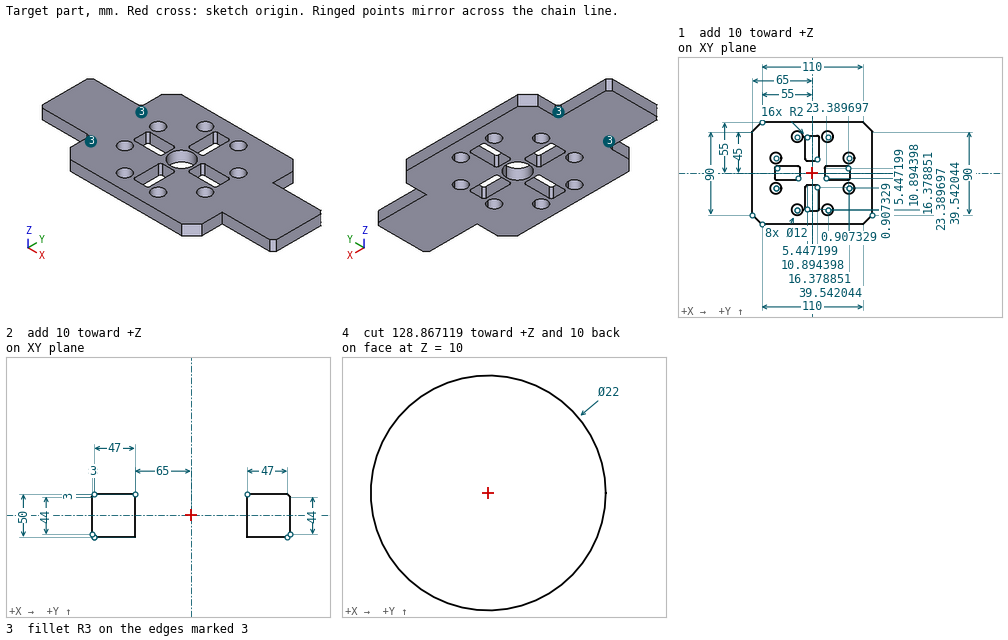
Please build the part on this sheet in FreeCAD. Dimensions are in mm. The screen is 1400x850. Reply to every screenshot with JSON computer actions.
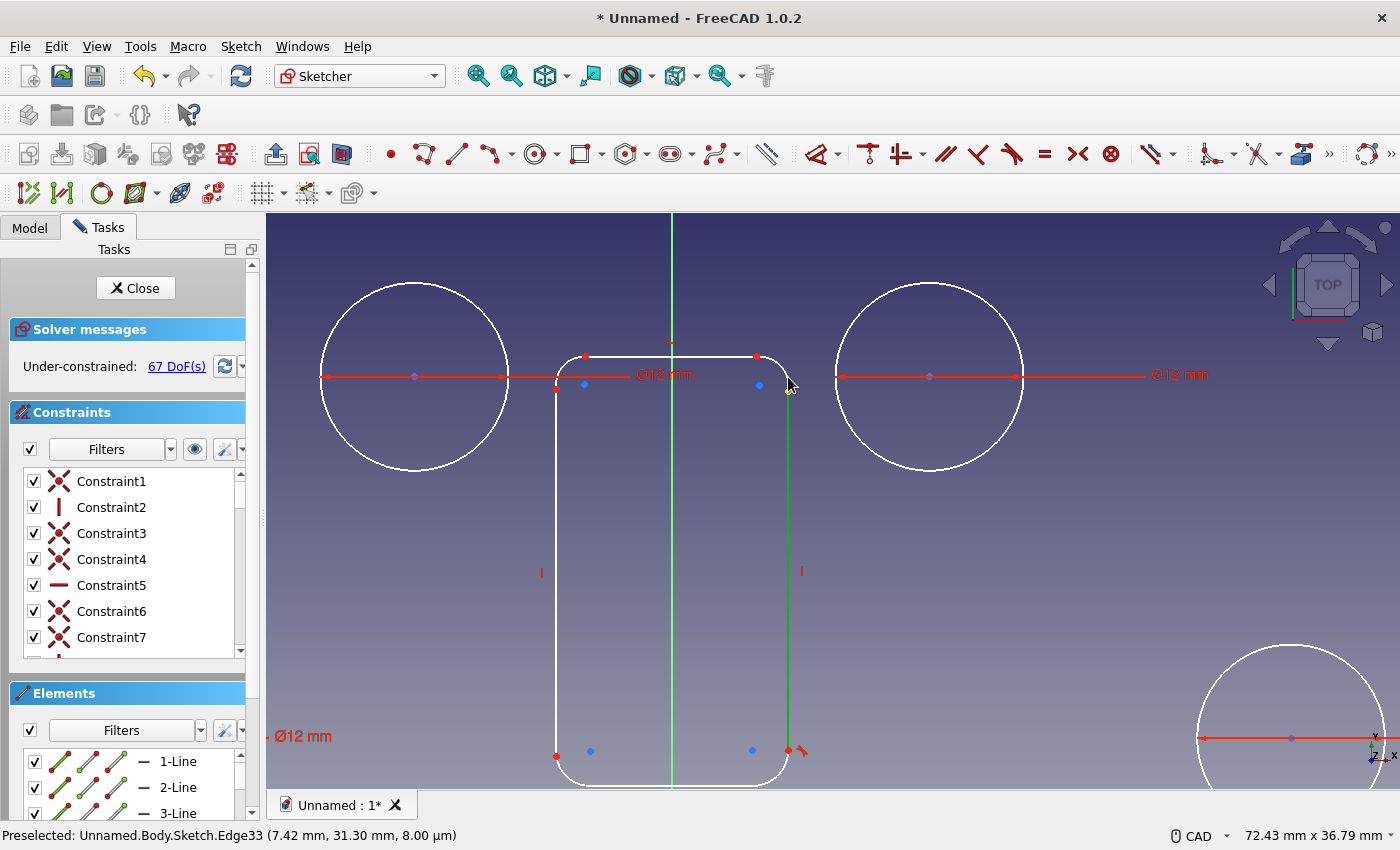
{"action": "left_click", "coordinate": [787, 375]}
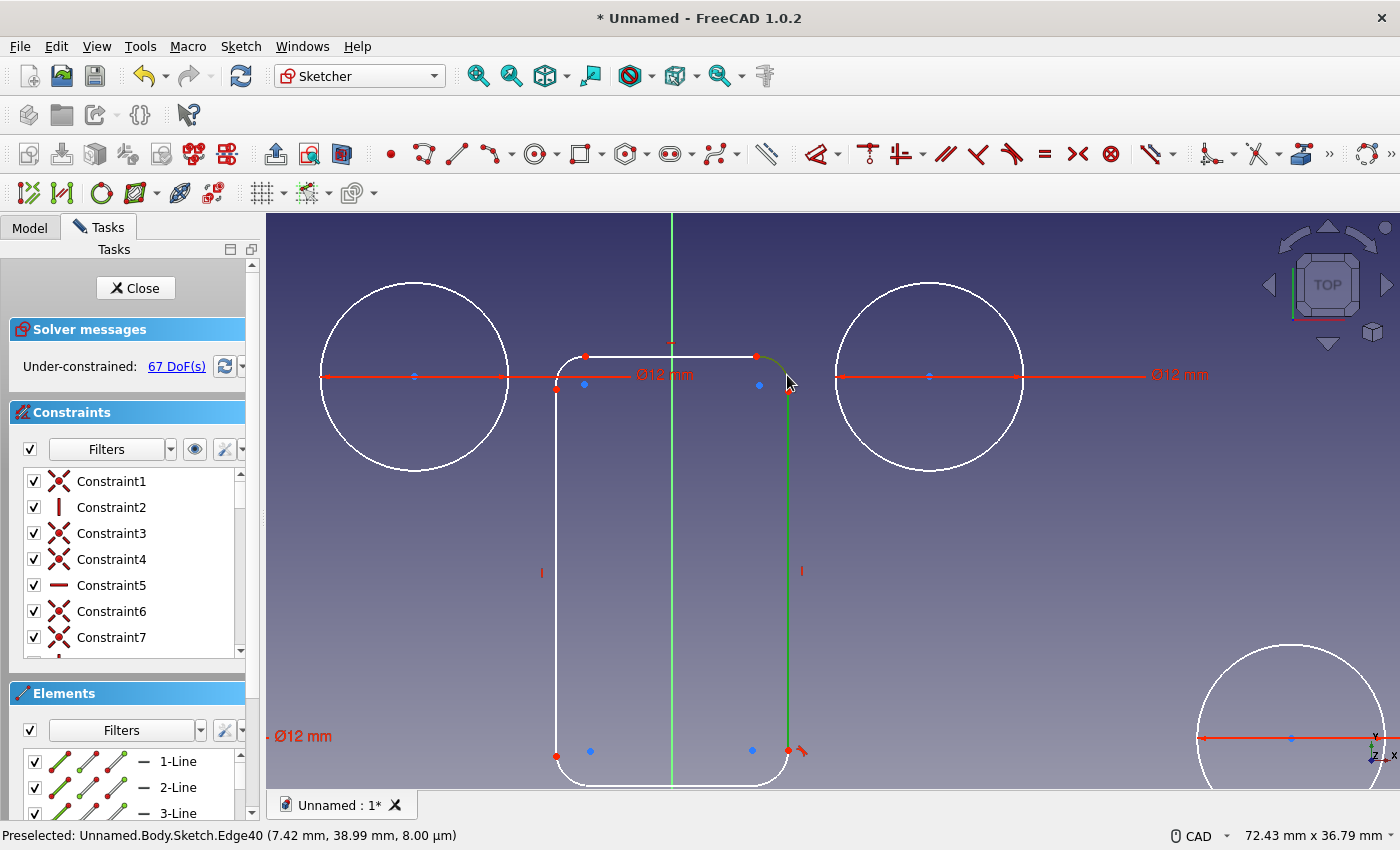
{"action": "left_click", "coordinate": [1012, 154]}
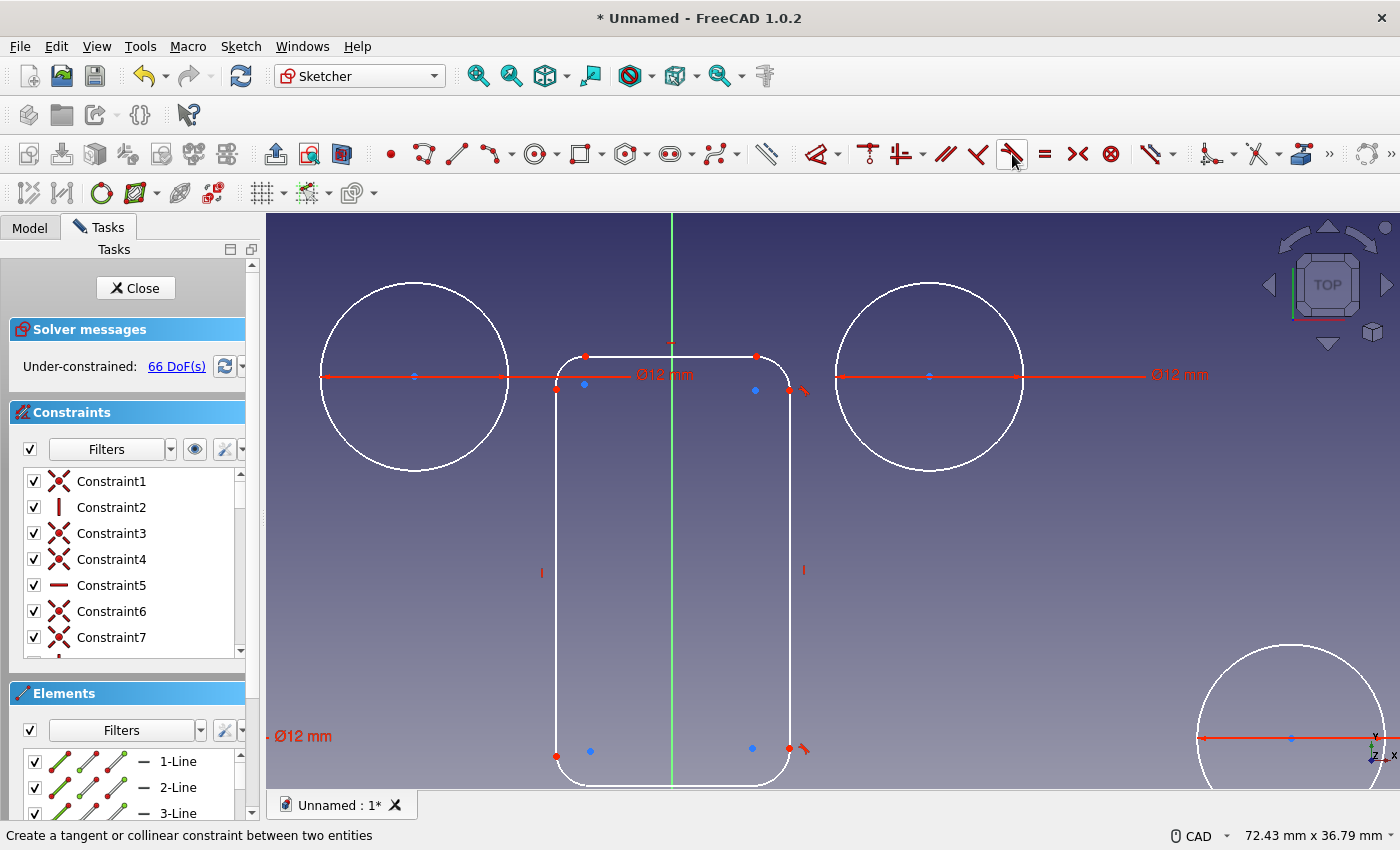
{"action": "scroll", "coordinate": [788, 377], "scroll_direction": "down", "scroll_amount": 8}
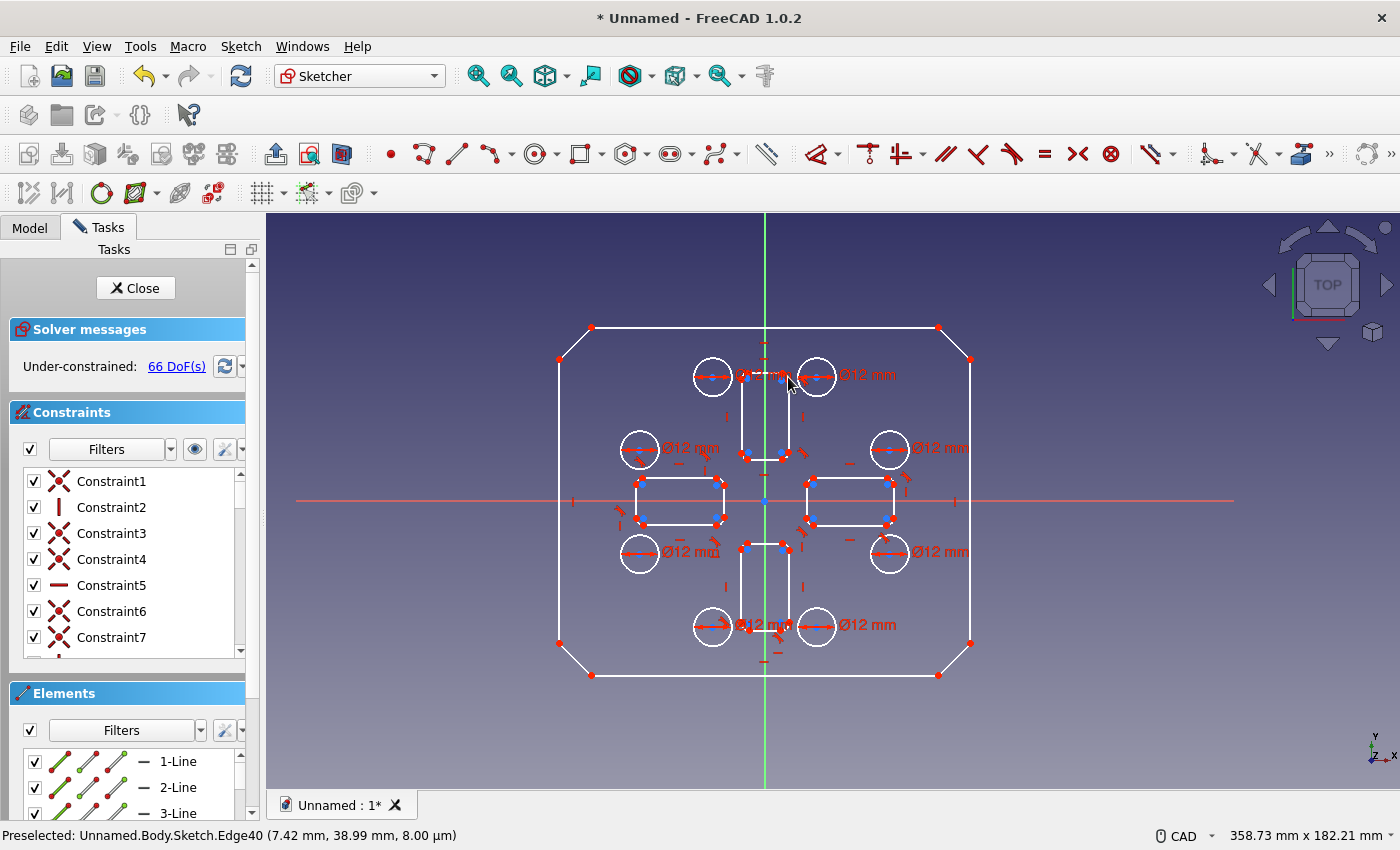
{"action": "scroll", "coordinate": [772, 460], "scroll_direction": "up", "scroll_amount": 4}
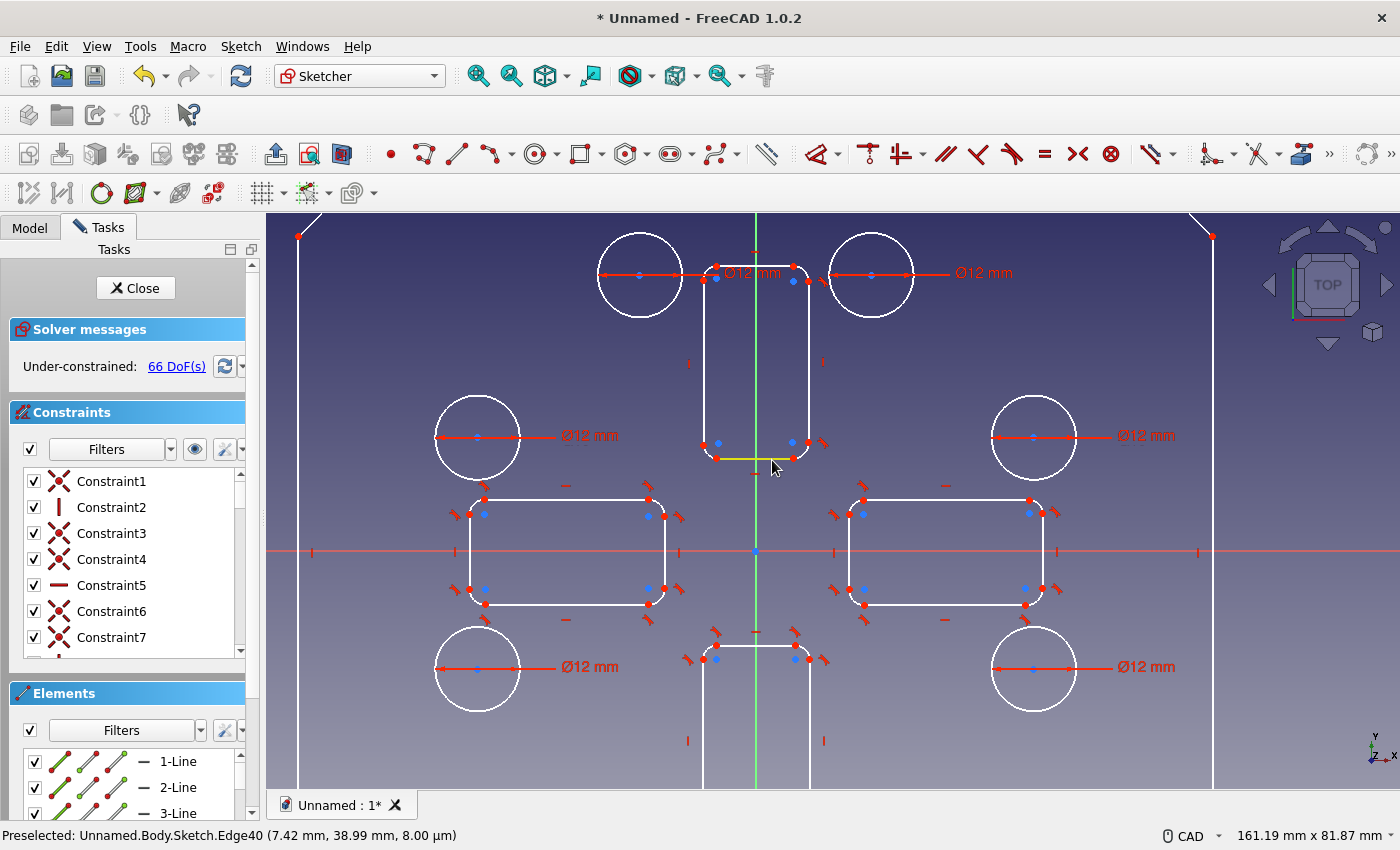
{"action": "left_click", "coordinate": [771, 459]}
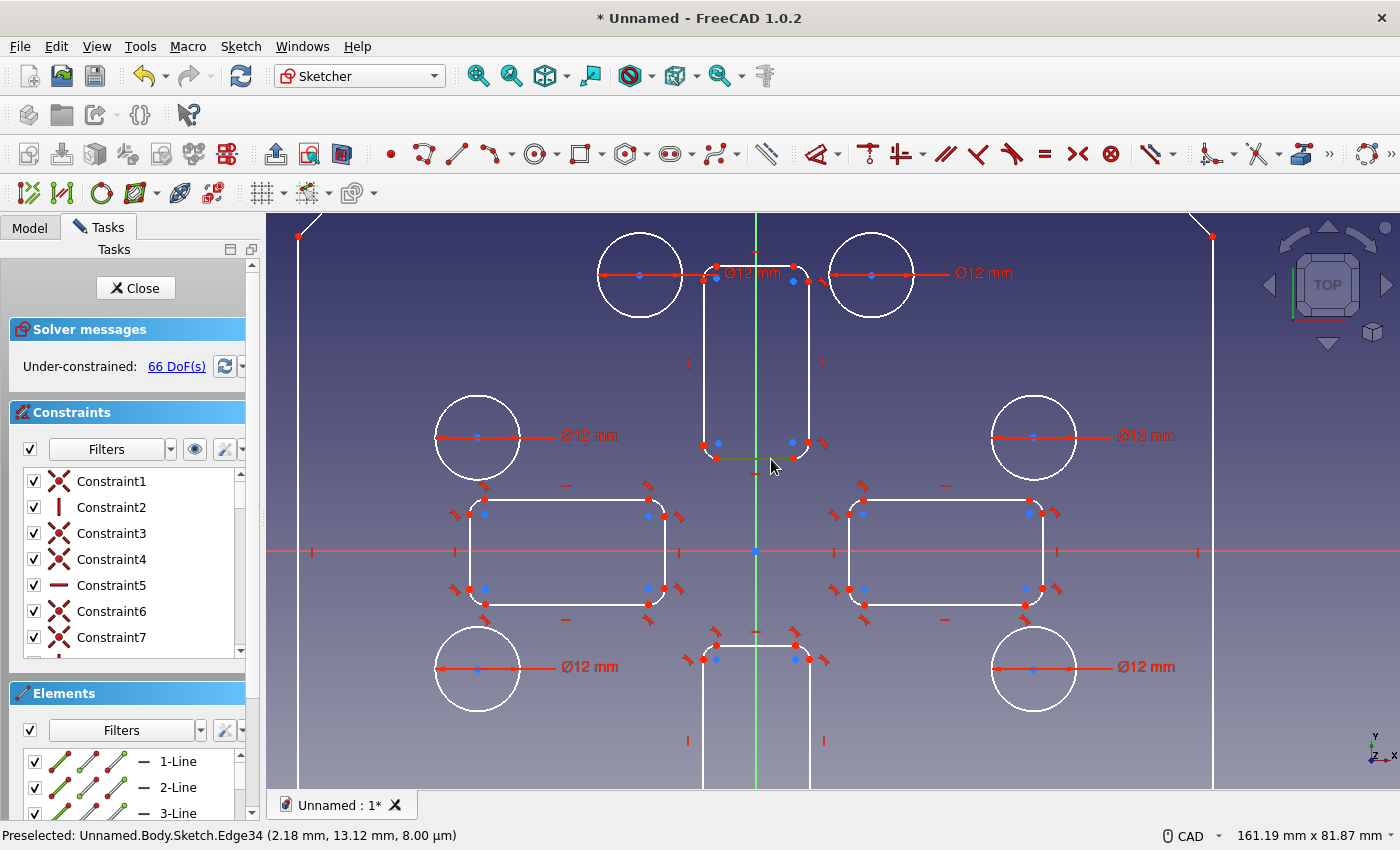
{"action": "left_click", "coordinate": [804, 453]}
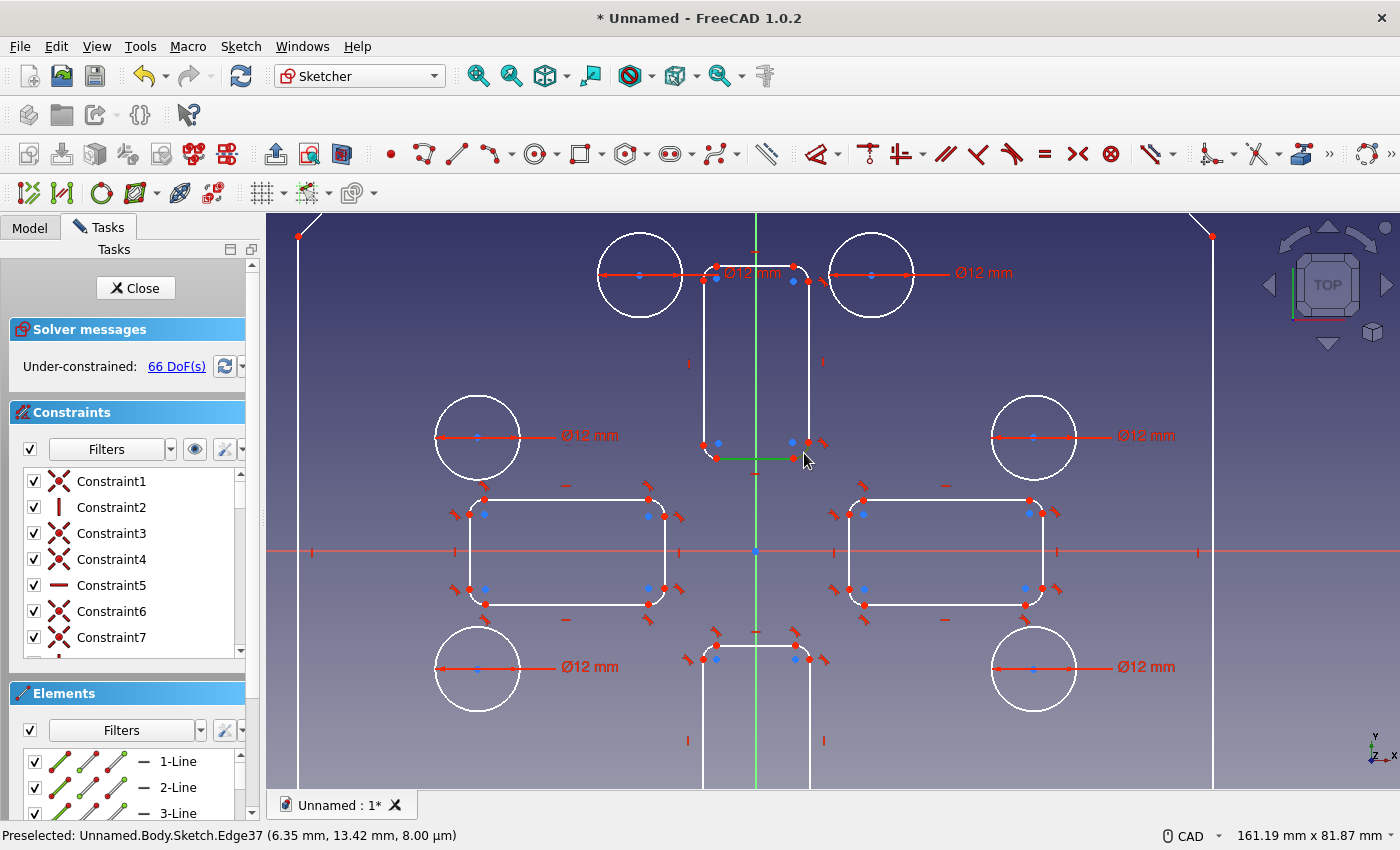
{"action": "left_click", "coordinate": [1012, 154]}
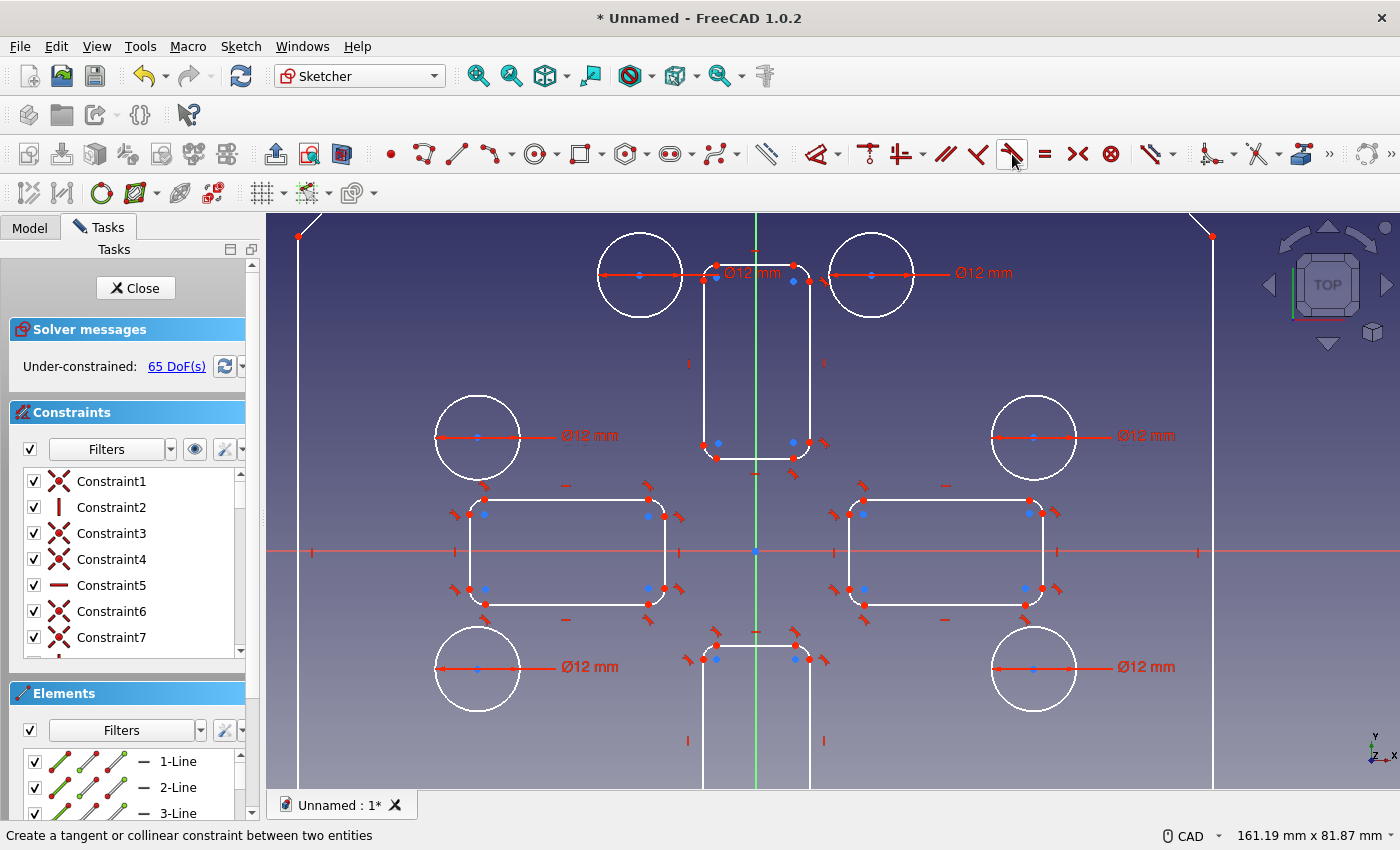
{"action": "left_click", "coordinate": [770, 459]}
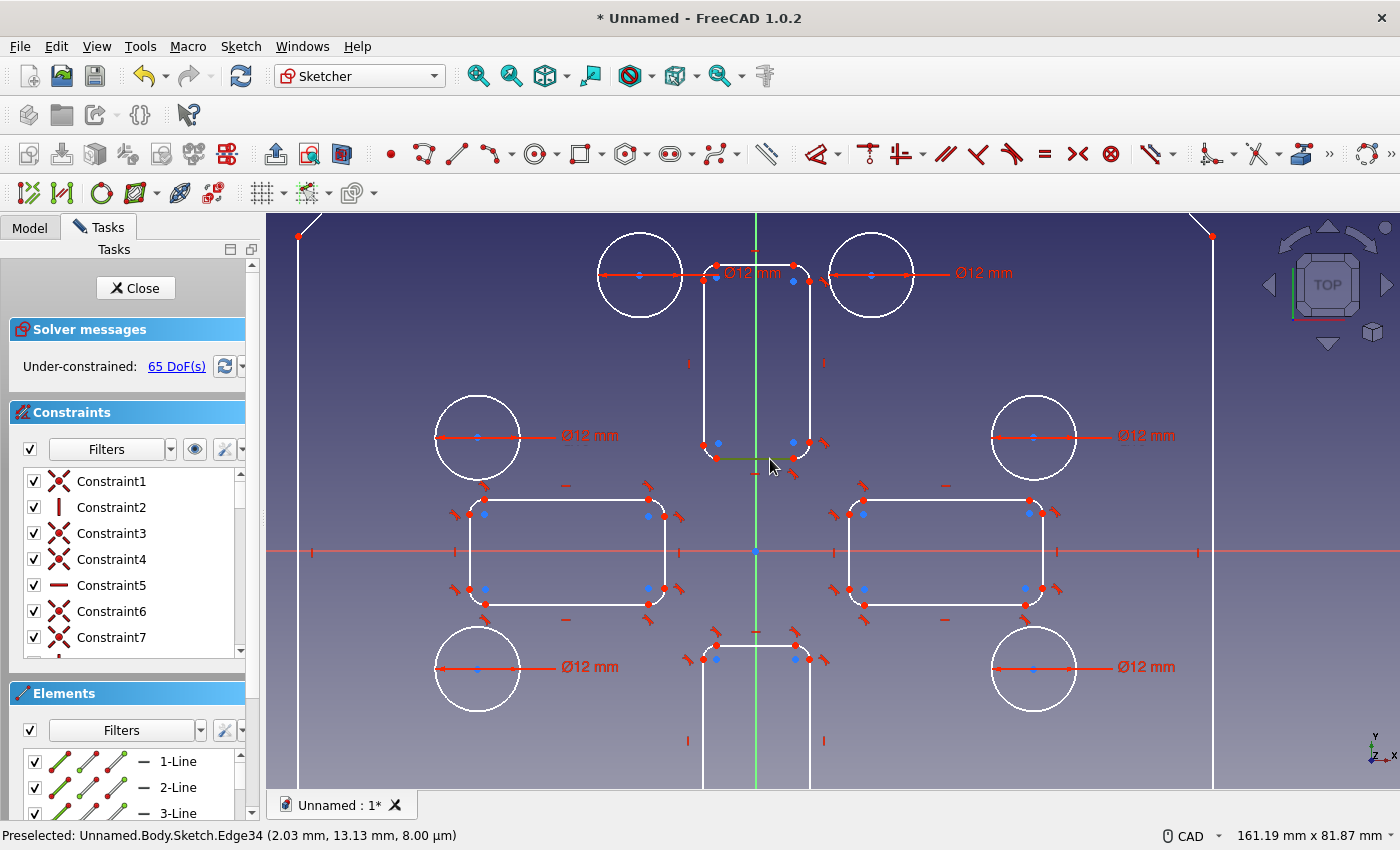
{"action": "scroll", "coordinate": [708, 454], "scroll_direction": "up", "scroll_amount": 2}